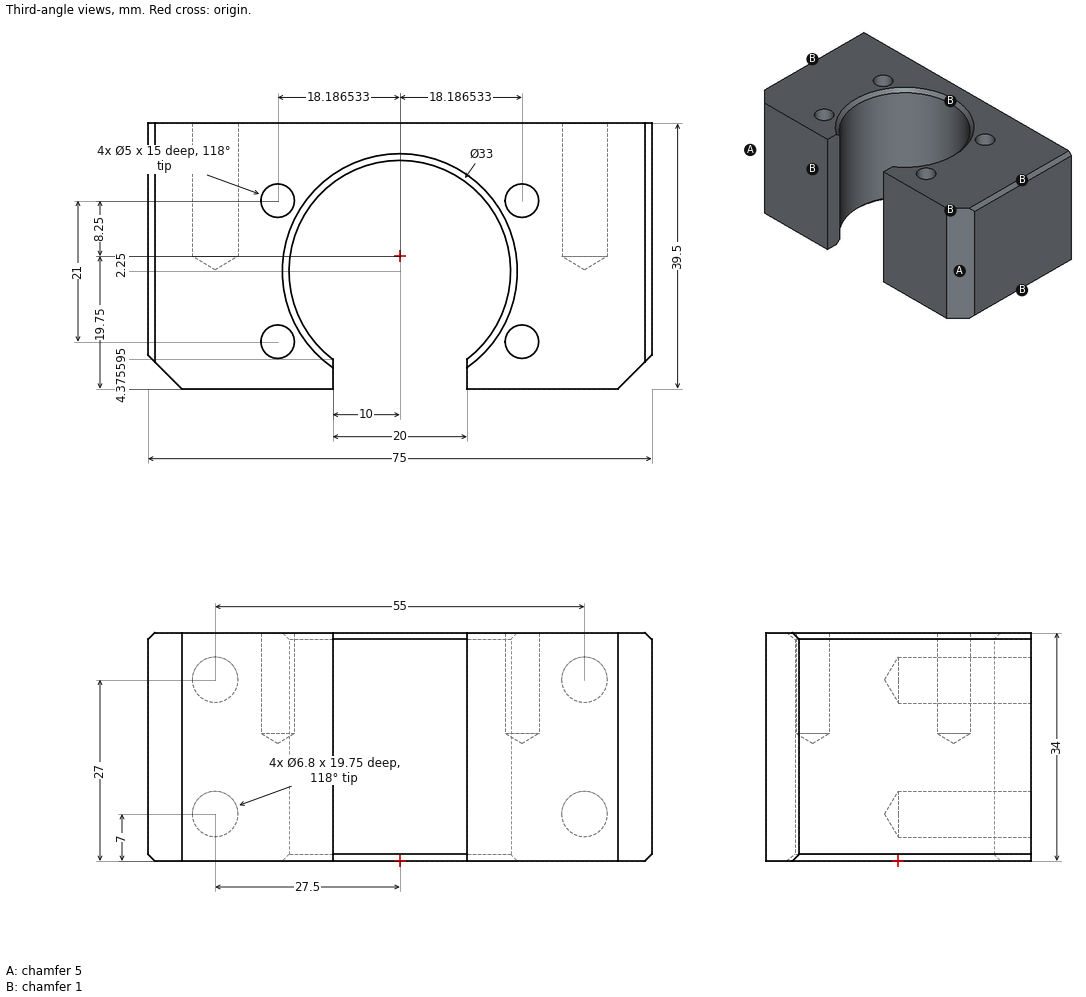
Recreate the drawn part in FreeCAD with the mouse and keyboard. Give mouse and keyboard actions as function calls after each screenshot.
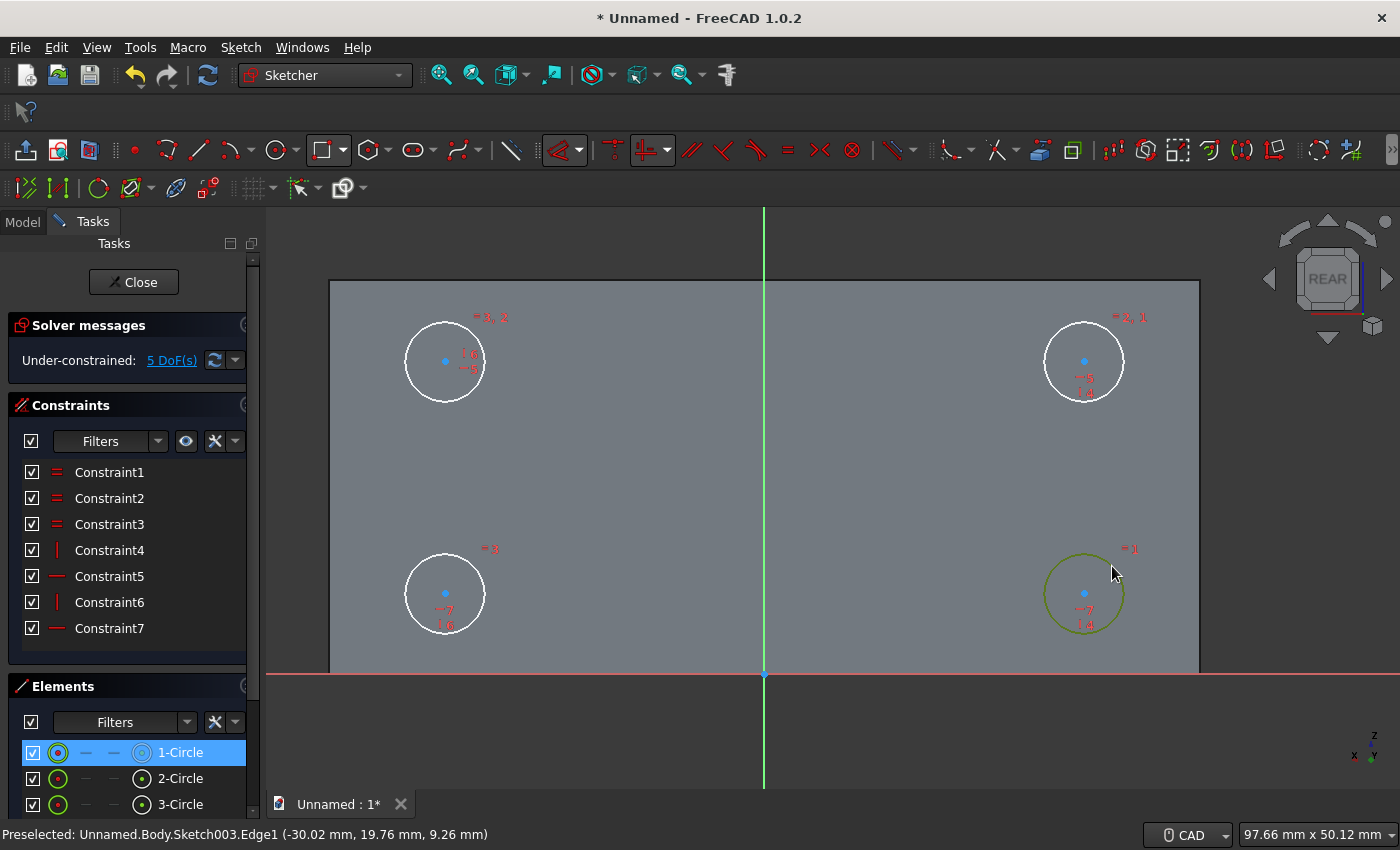
click(582, 150)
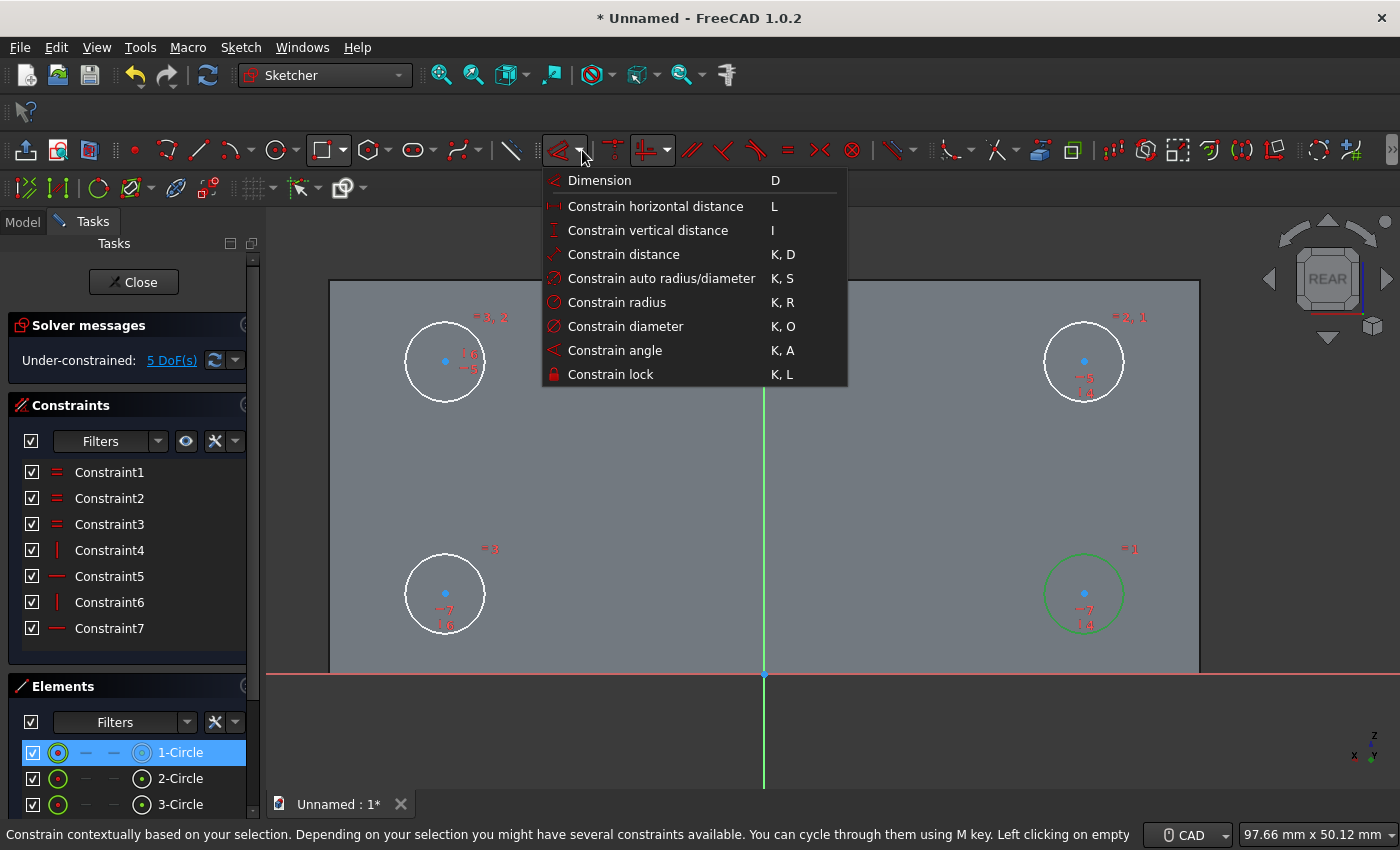
click(695, 326)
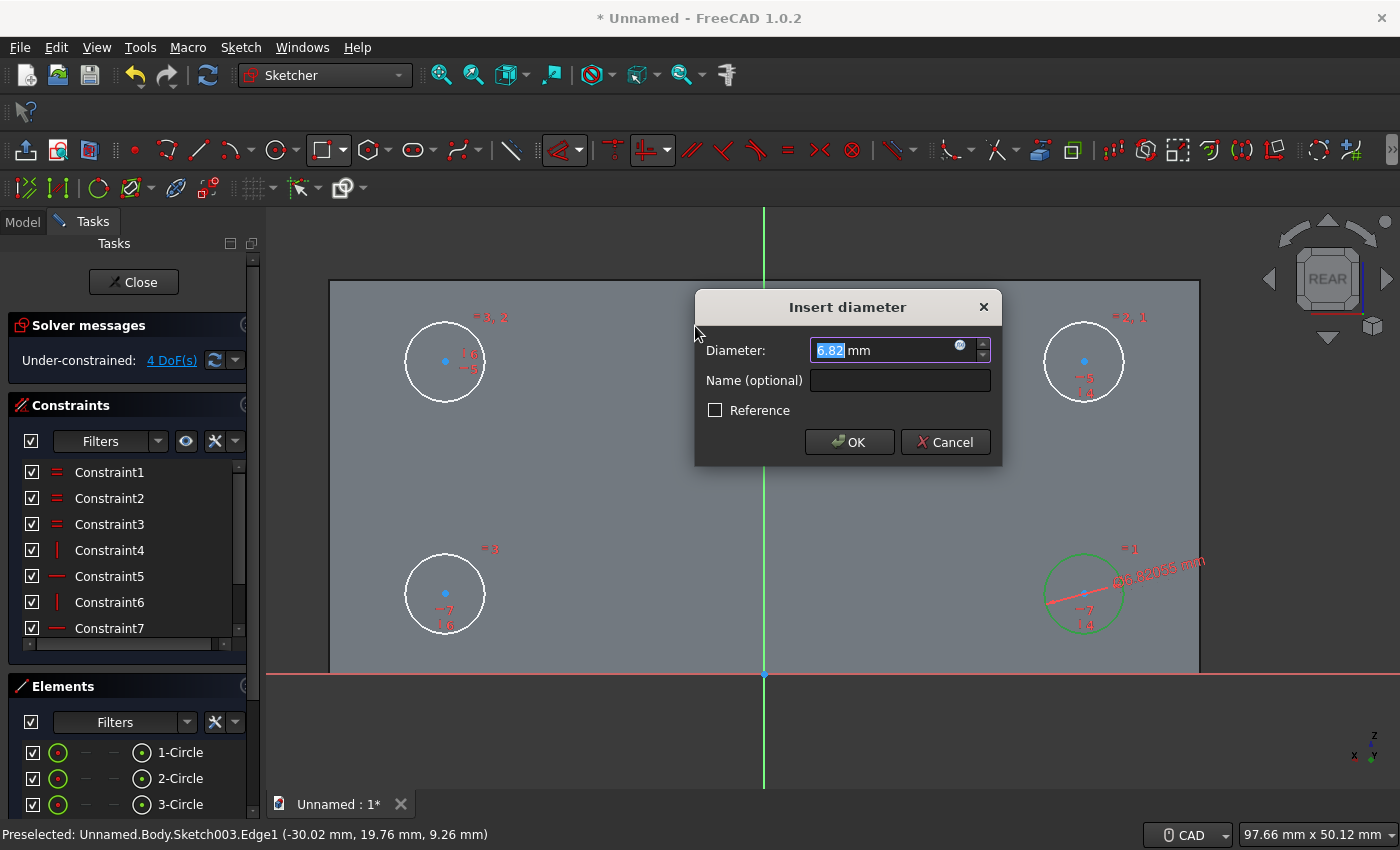
text(6.8)
key(Return)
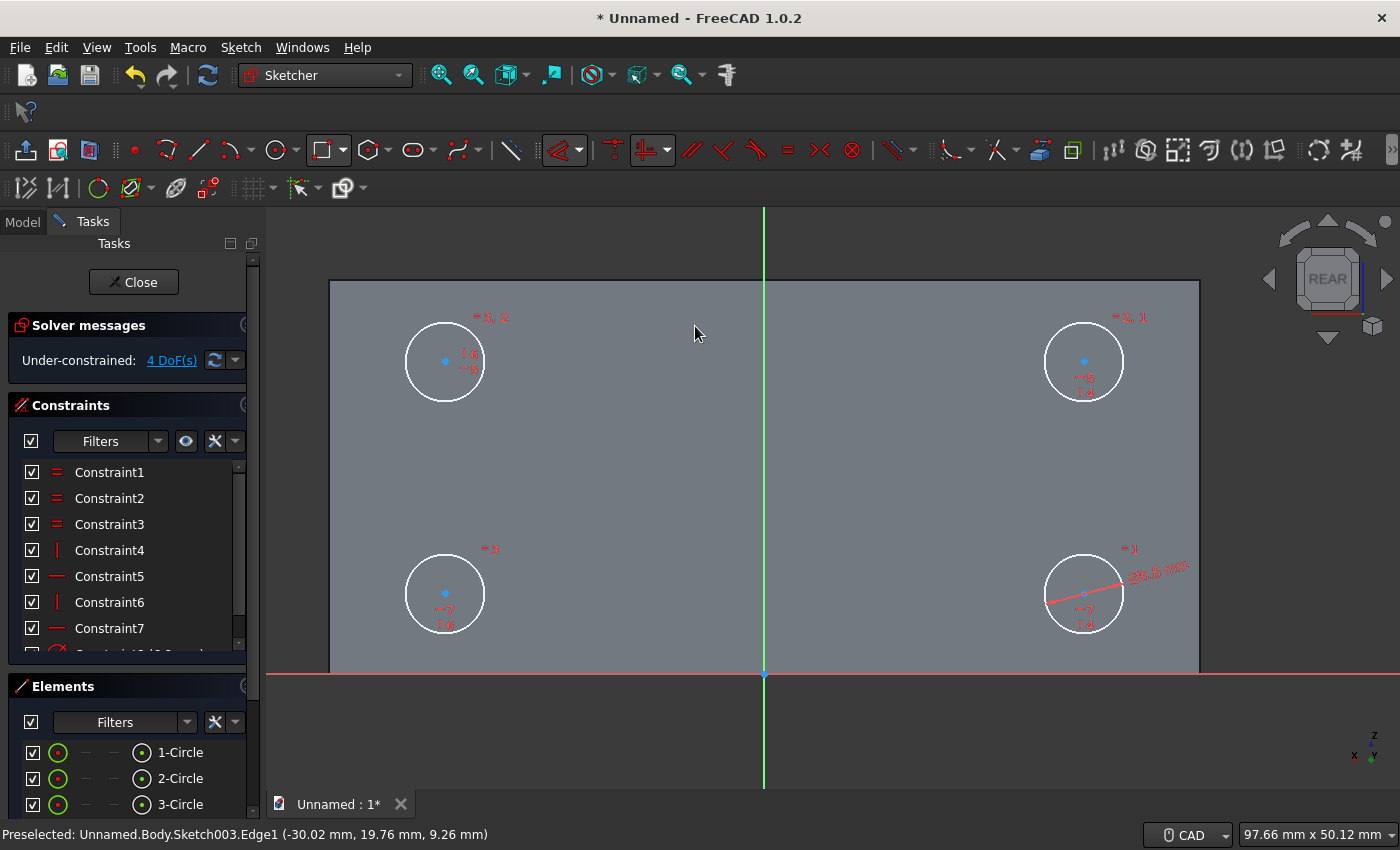
click(1084, 594)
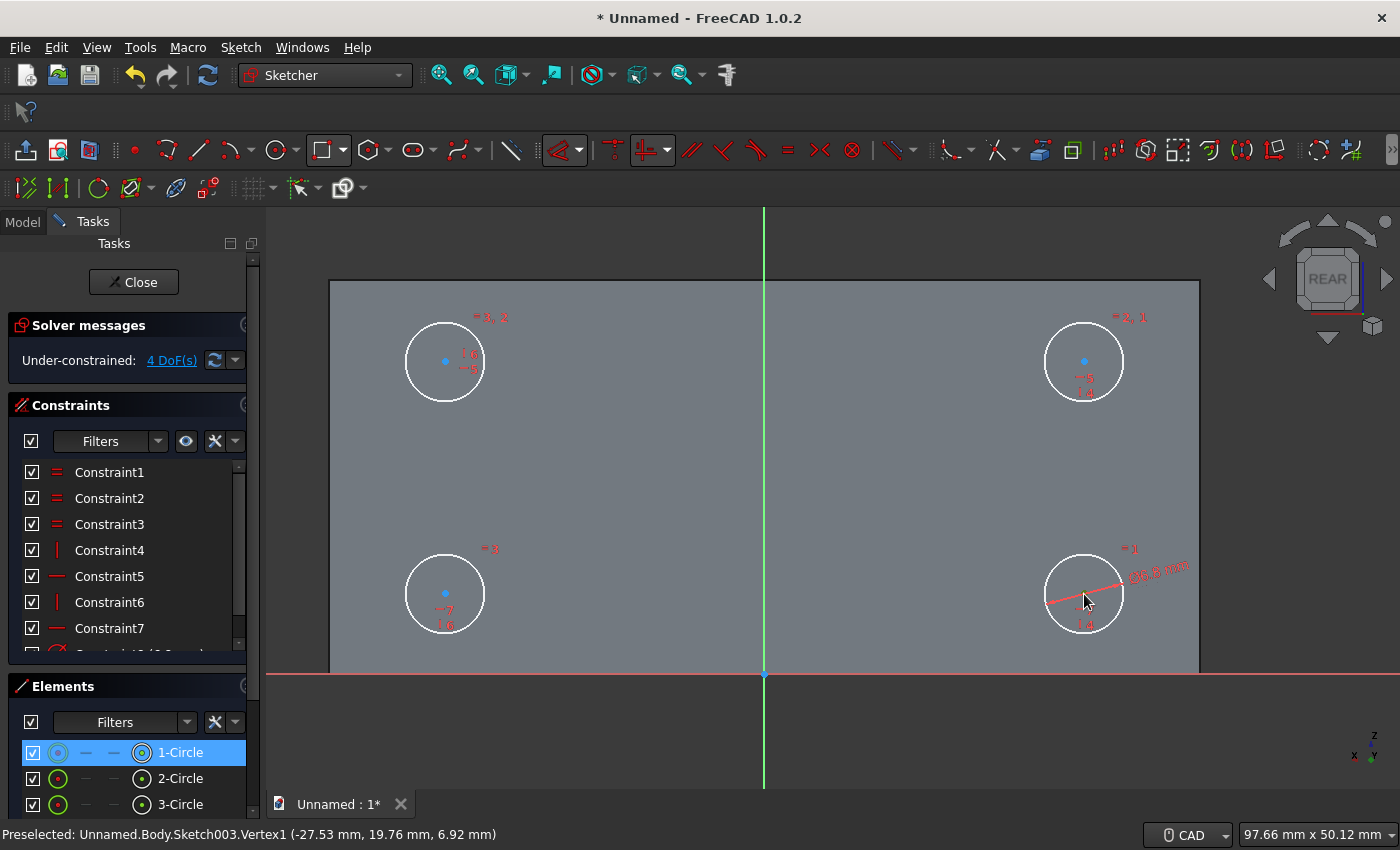
click(582, 150)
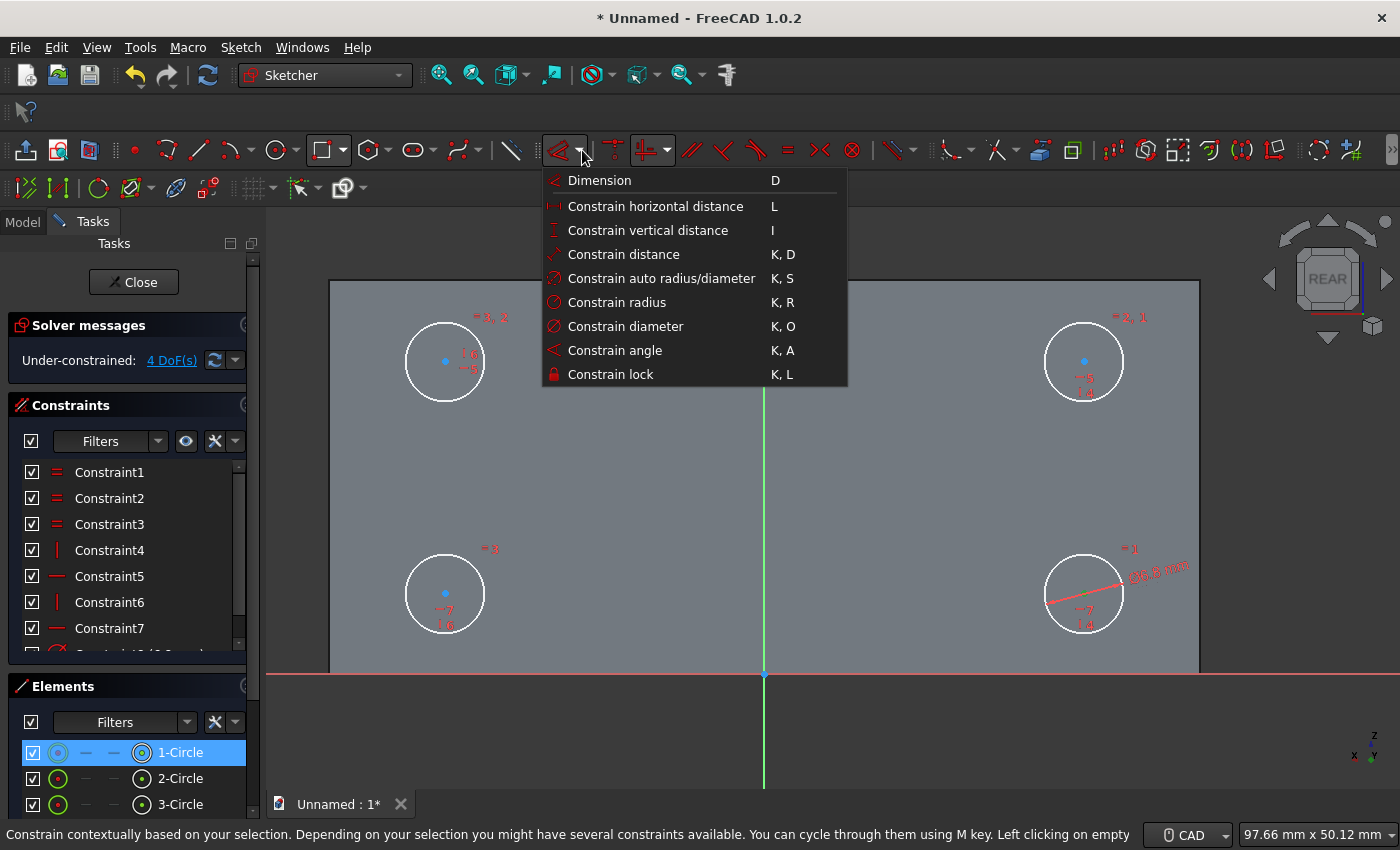
click(695, 230)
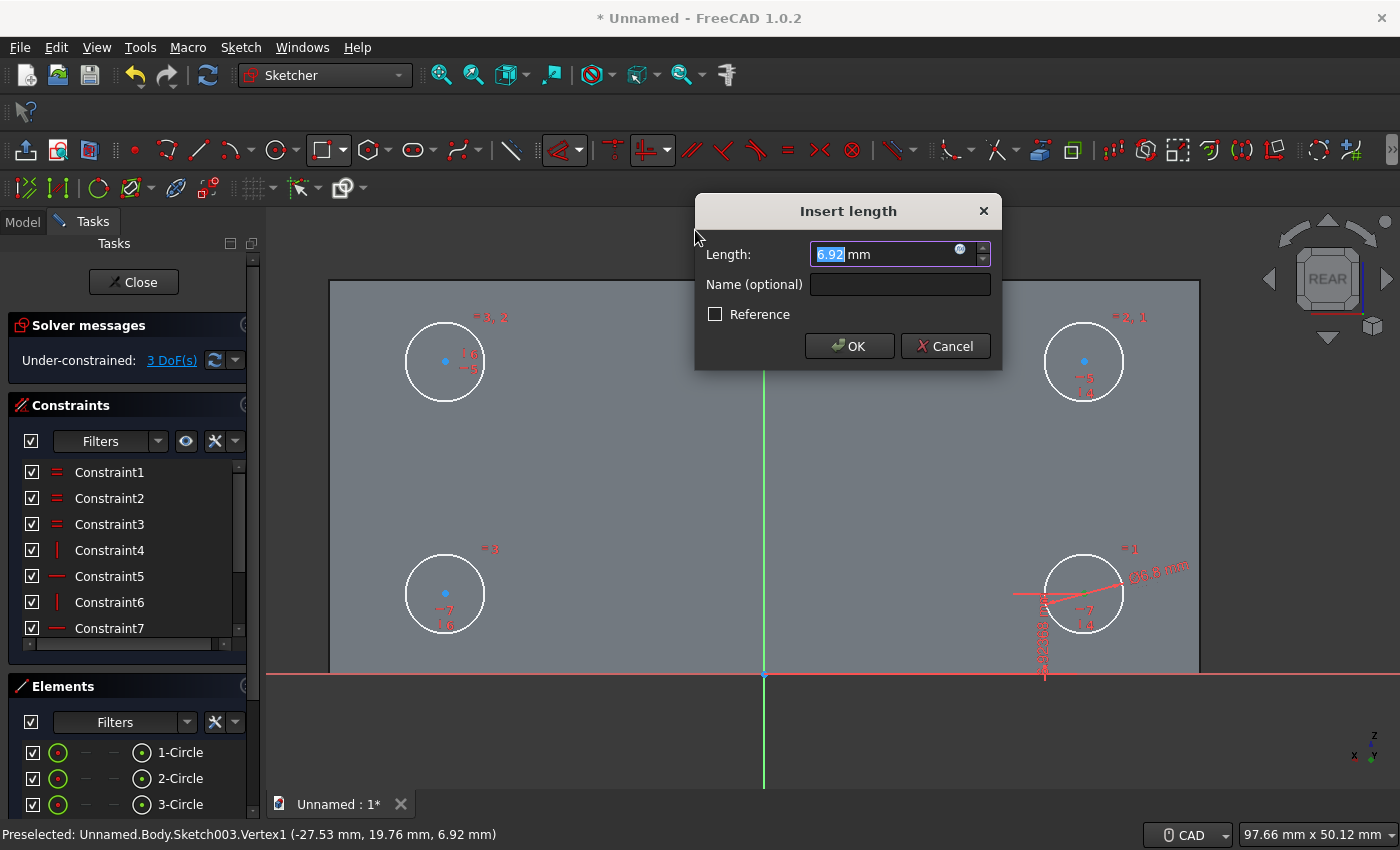
text(7)
key(Return)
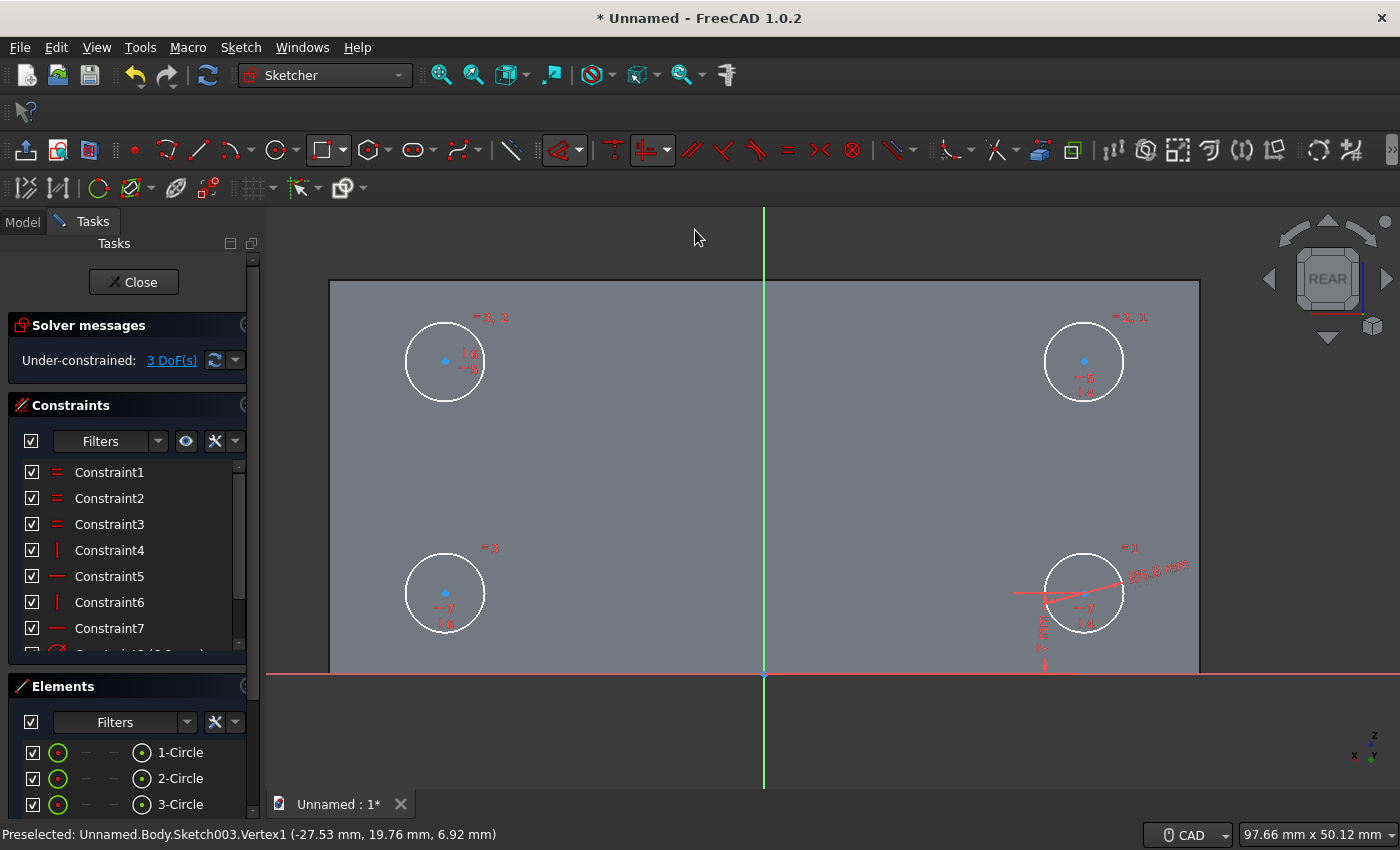
click(1084, 362)